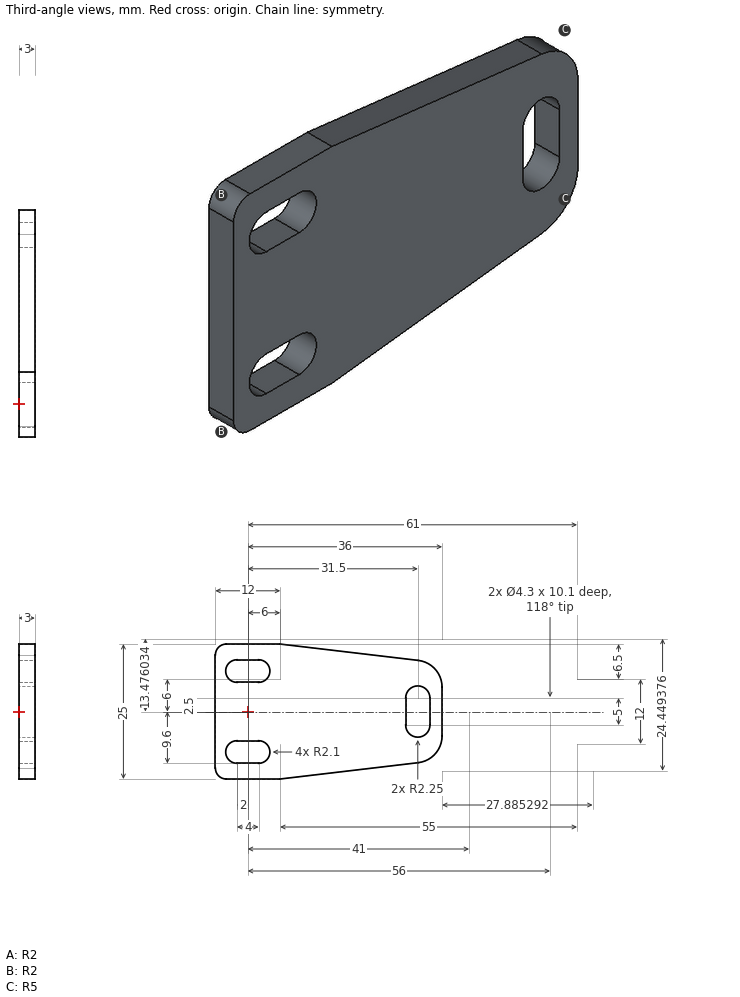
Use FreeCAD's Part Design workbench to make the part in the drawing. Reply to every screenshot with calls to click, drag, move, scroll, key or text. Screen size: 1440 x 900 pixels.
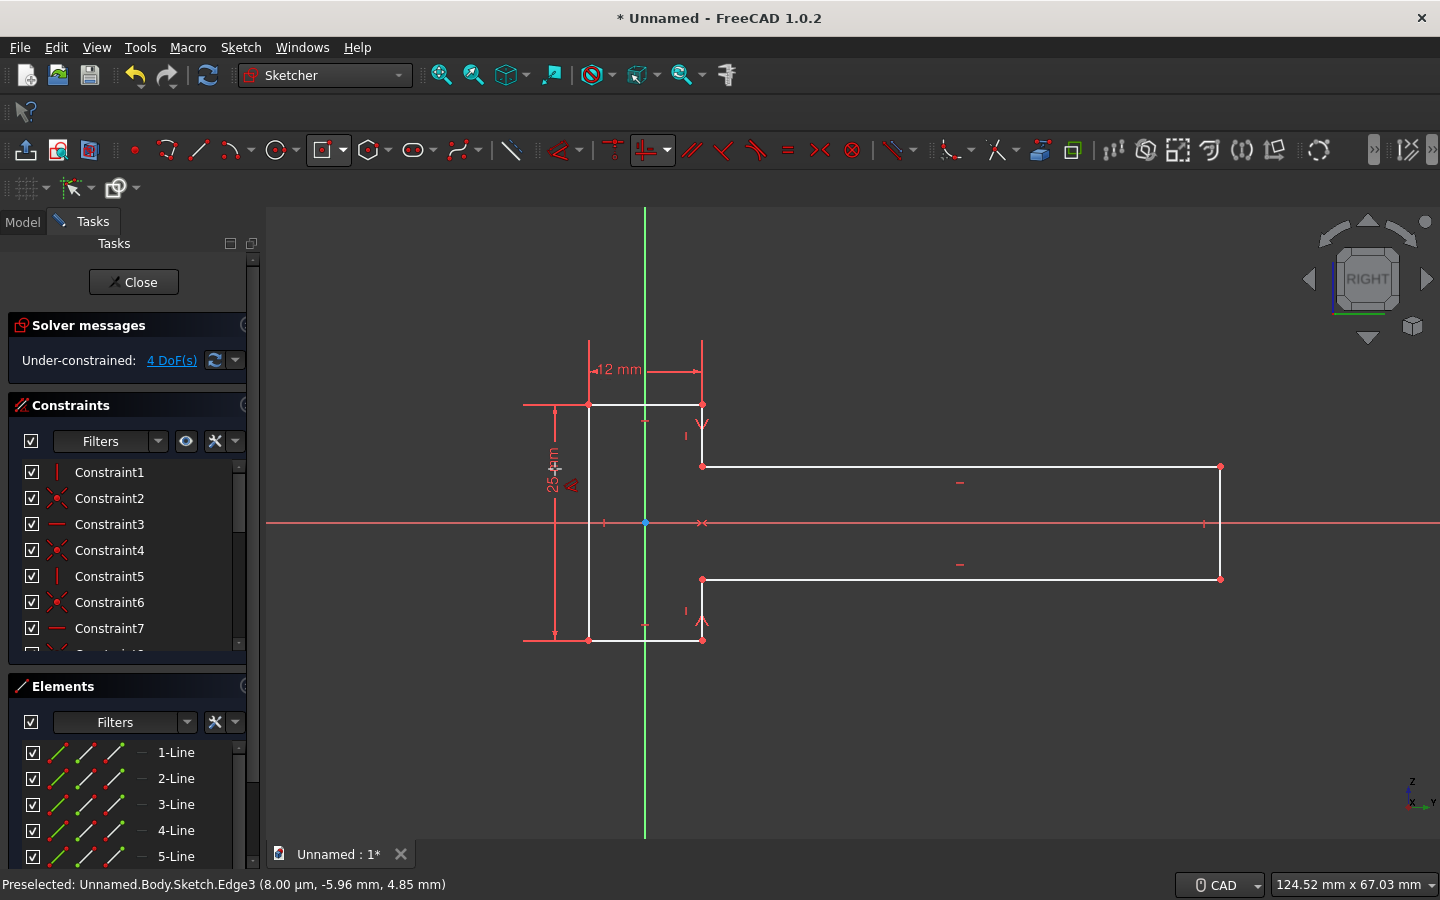
click(857, 580)
click(961, 614)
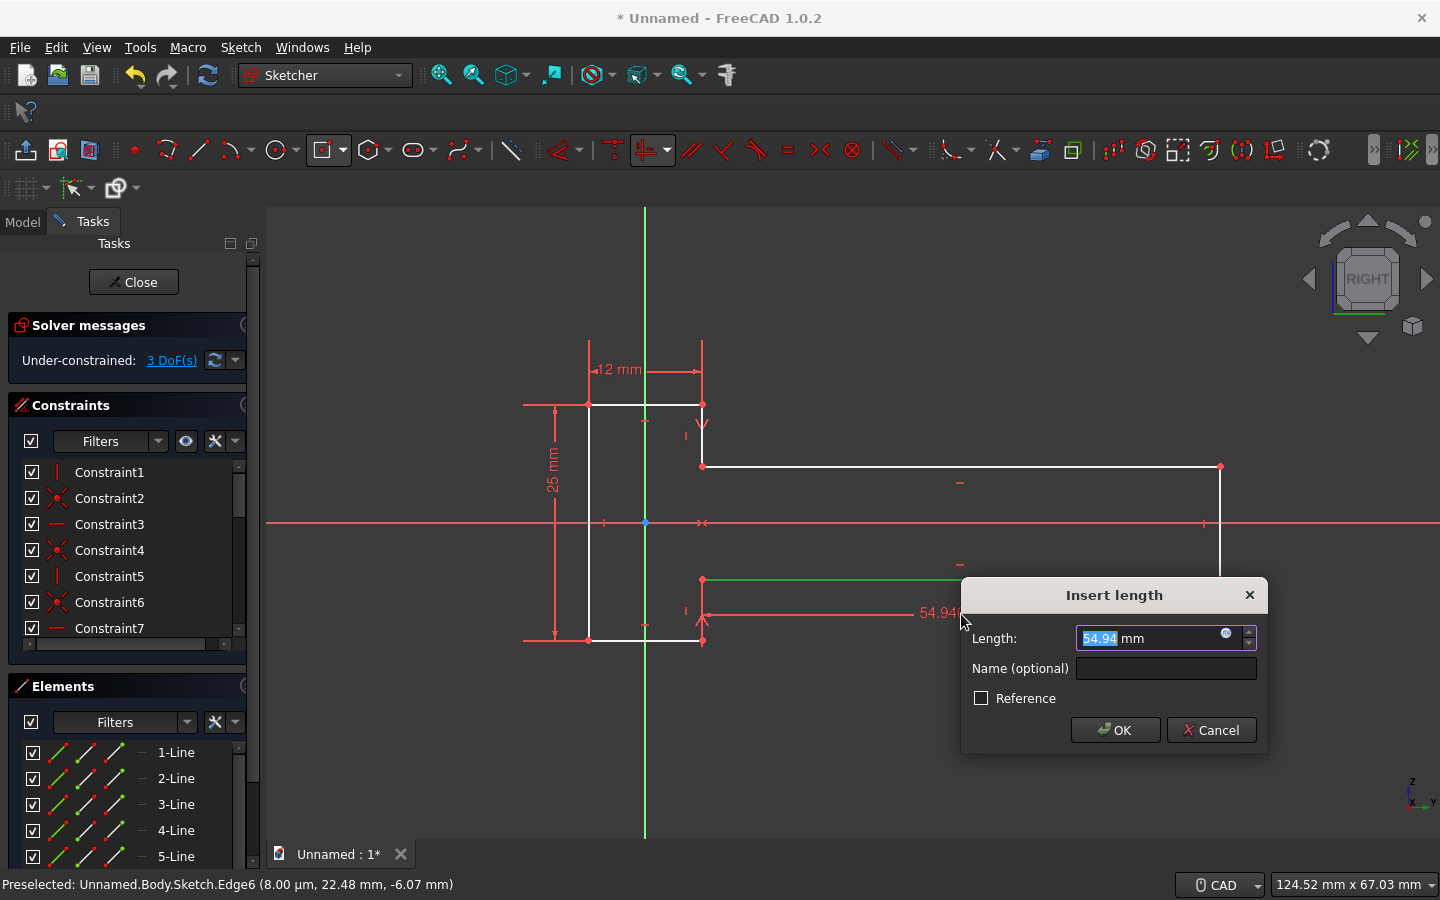
text(55)
key(Return)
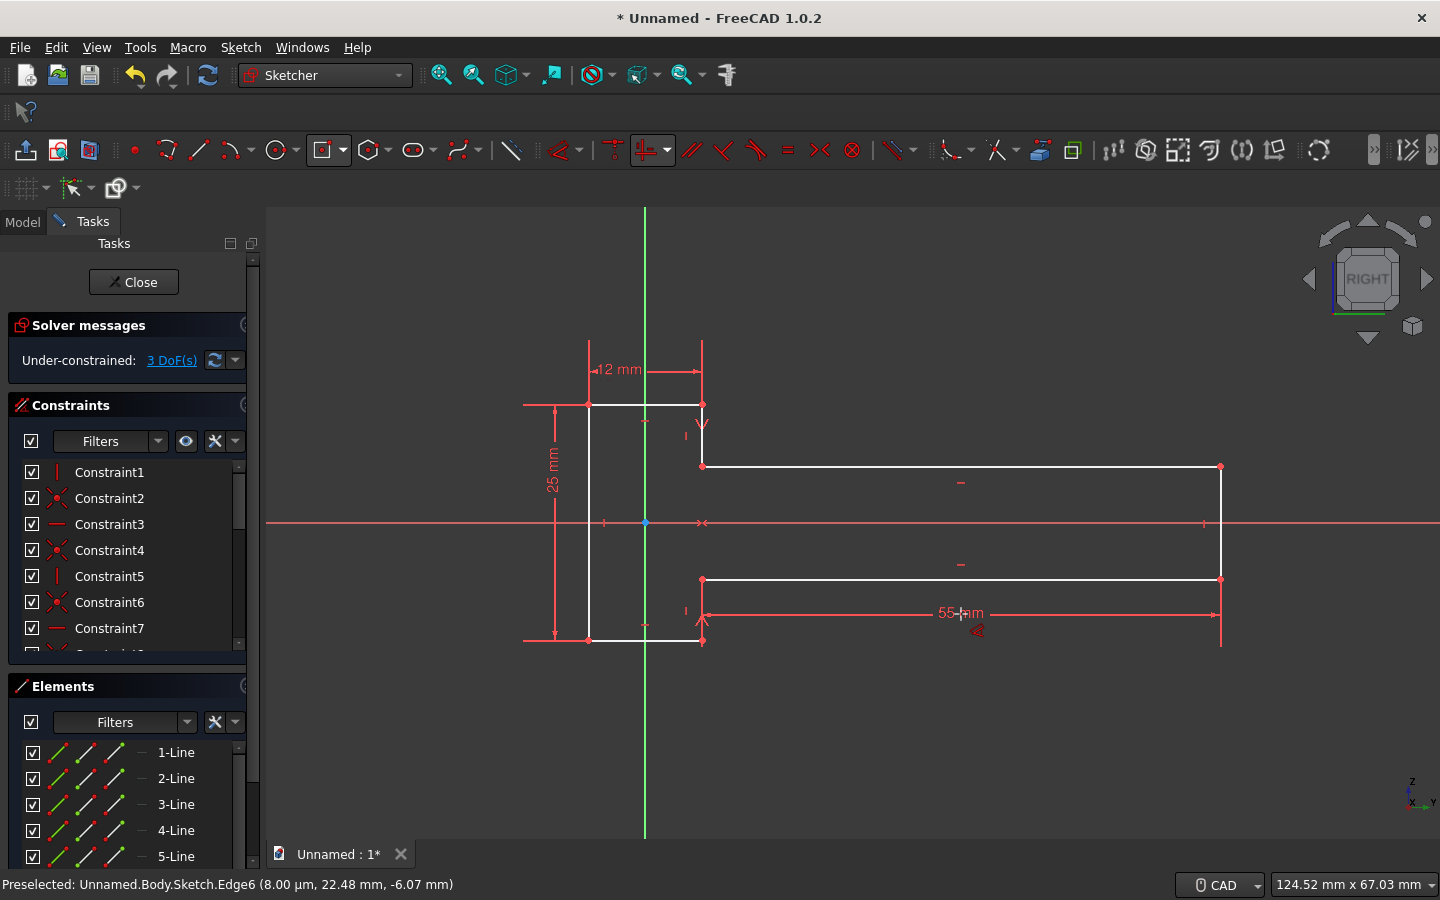
click(1221, 546)
click(1255, 498)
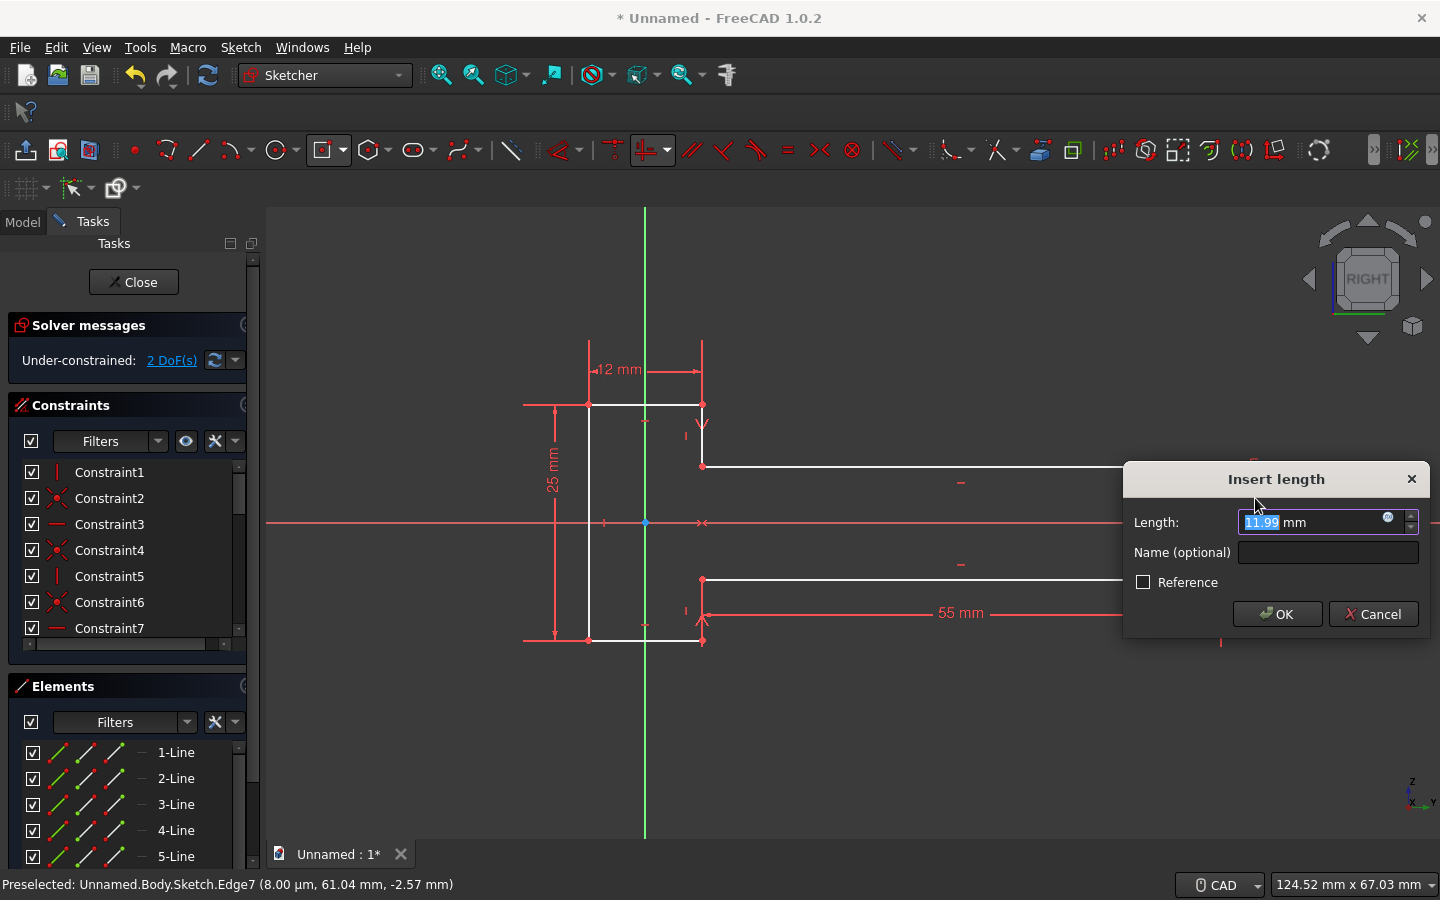
text(12)
key(Return)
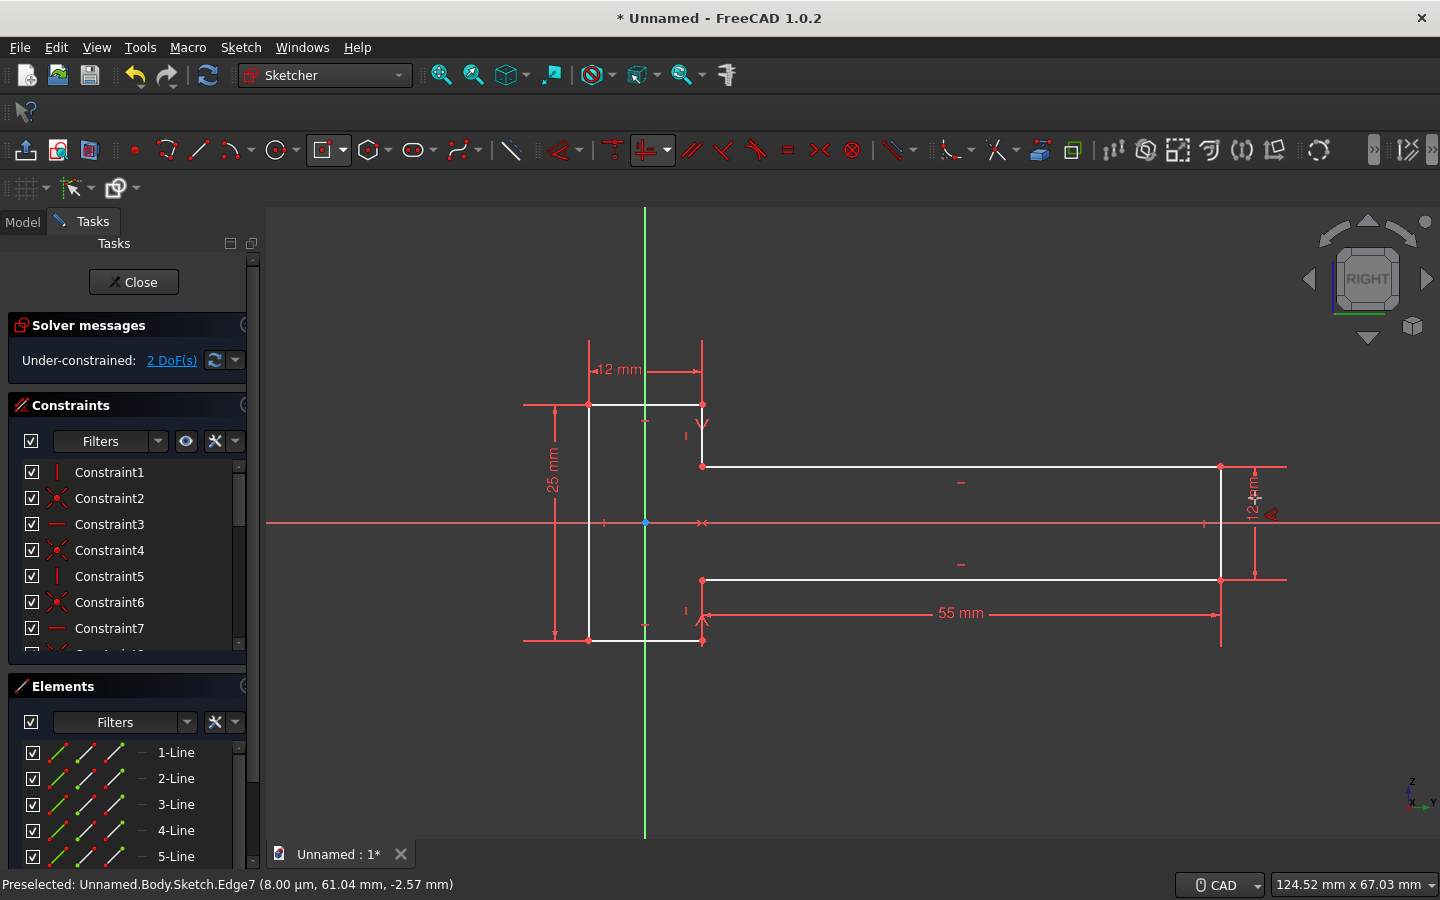
click(702, 467)
click(674, 433)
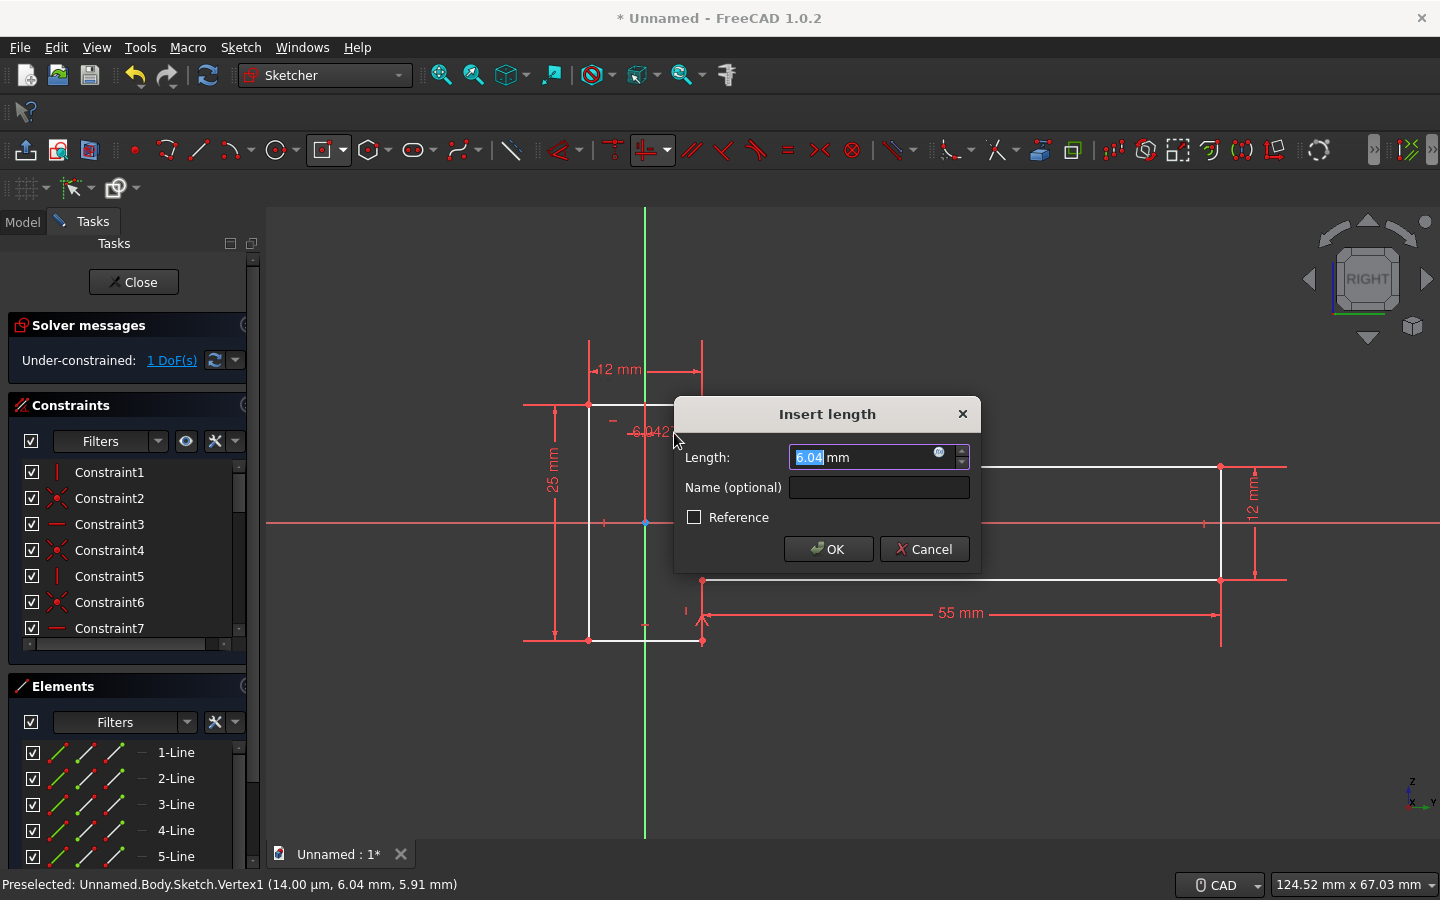
text(6)
key(Return)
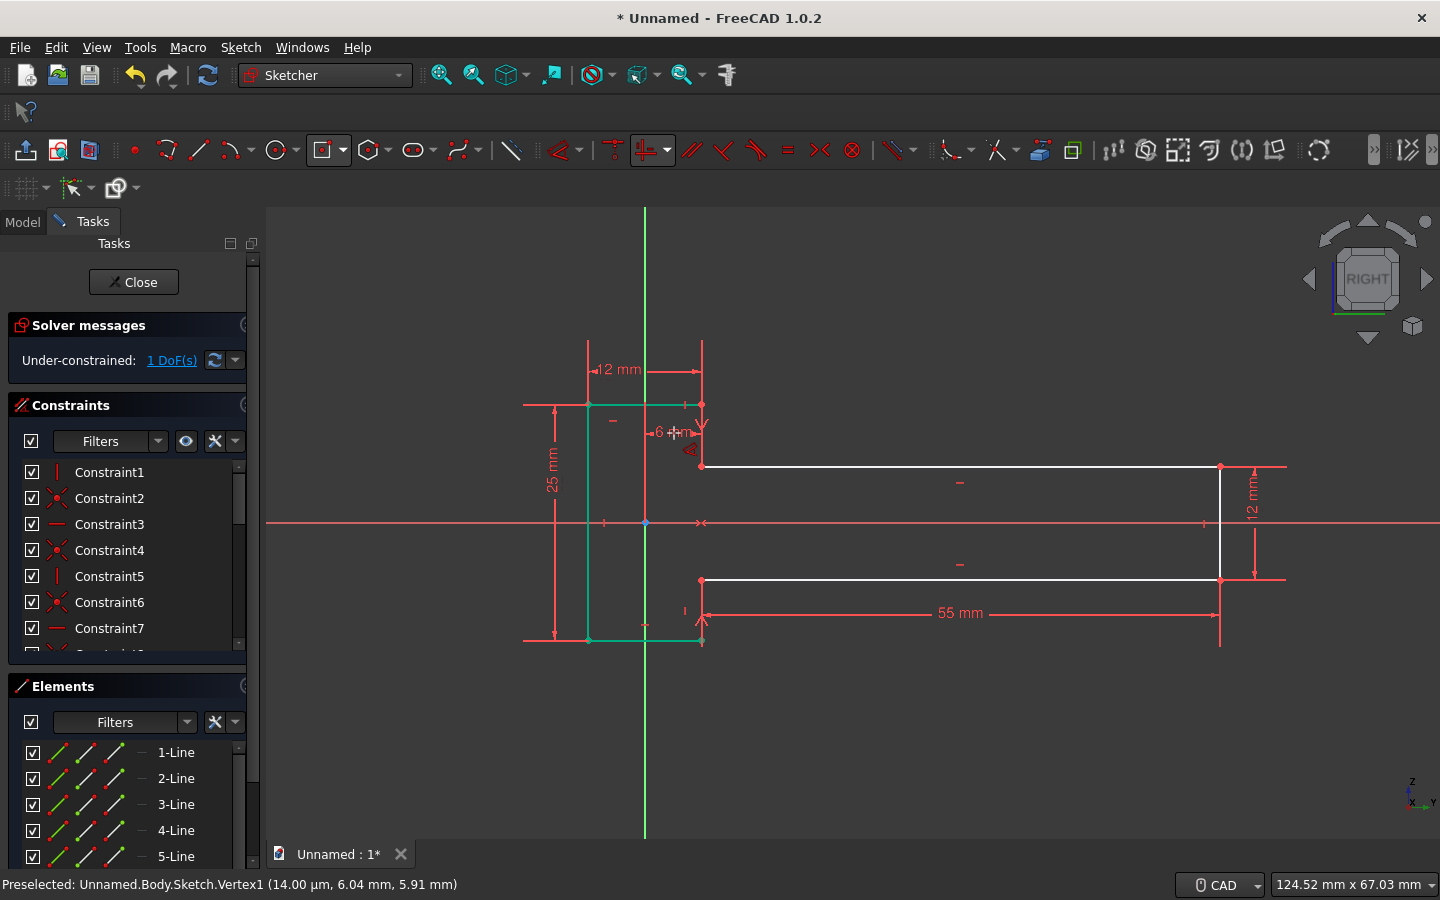
click(702, 467)
click(611, 495)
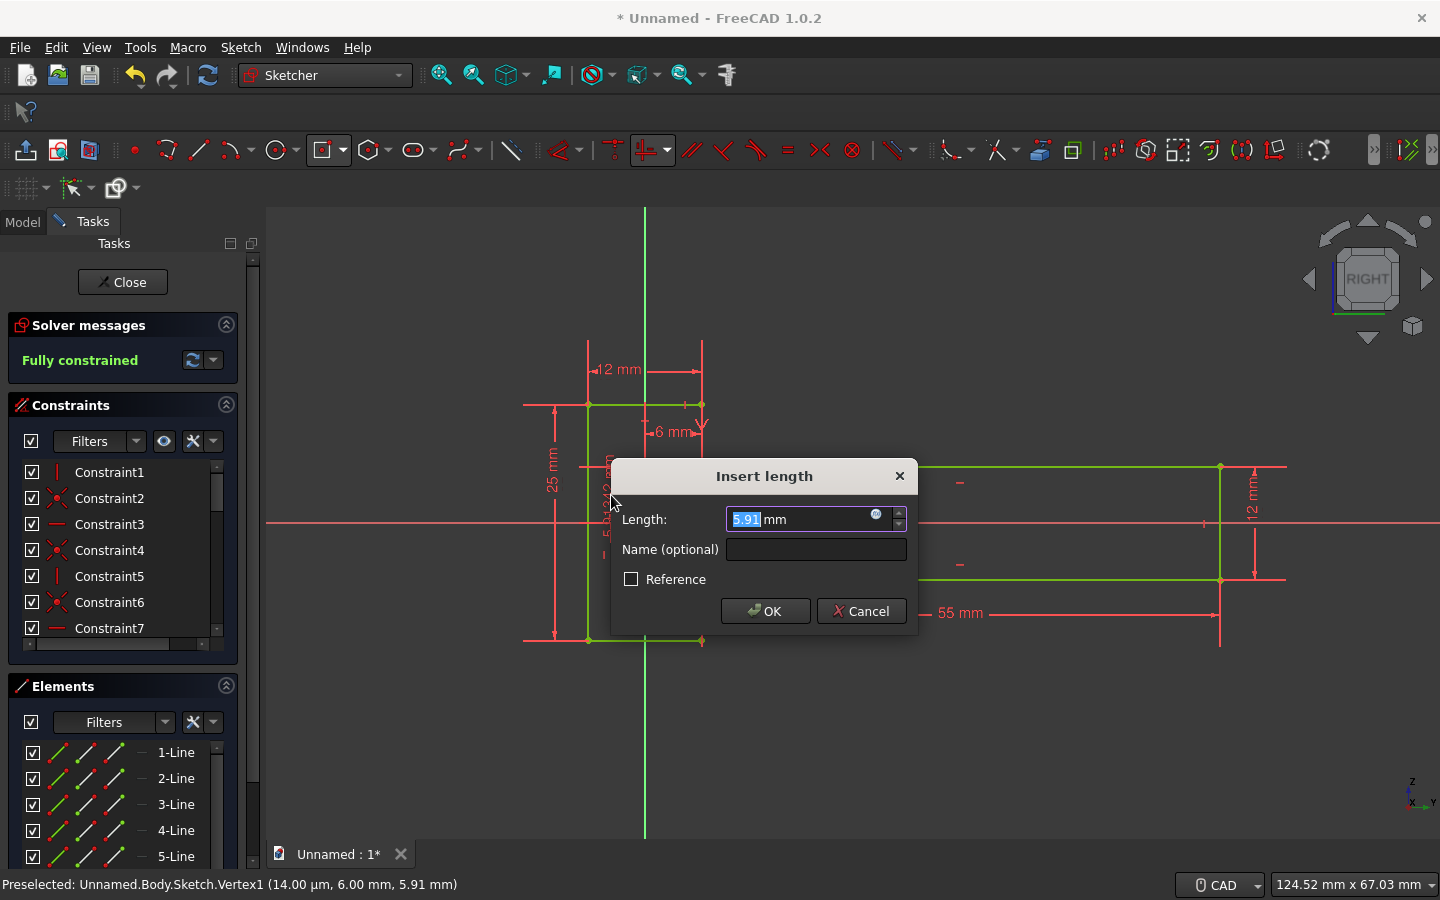
text(6)
key(Return)
key(Escape)